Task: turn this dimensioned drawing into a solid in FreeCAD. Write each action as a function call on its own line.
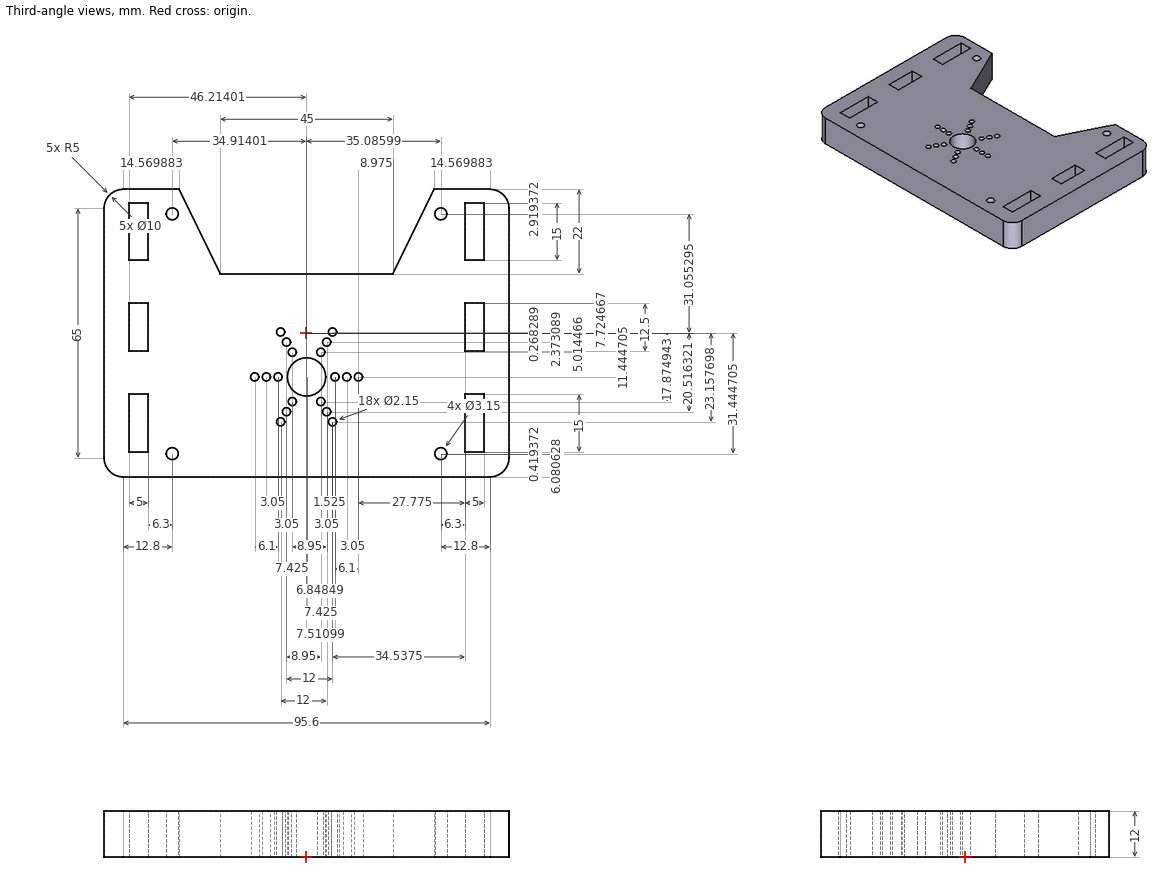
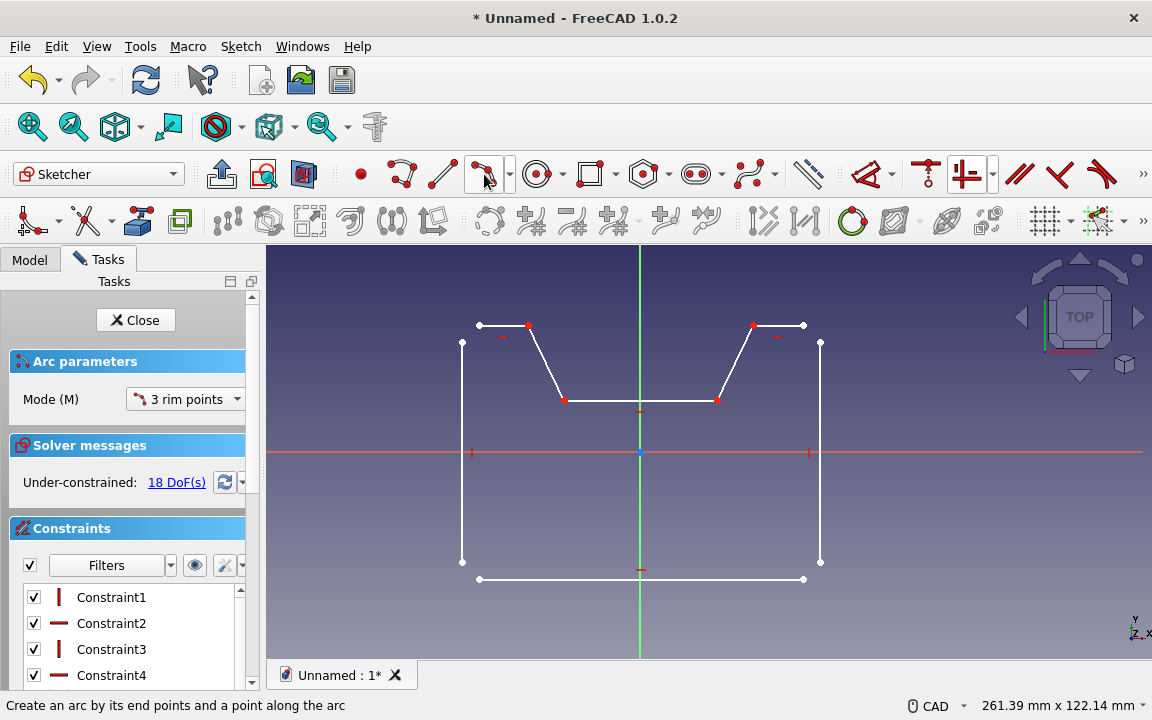
click(462, 563)
click(479, 580)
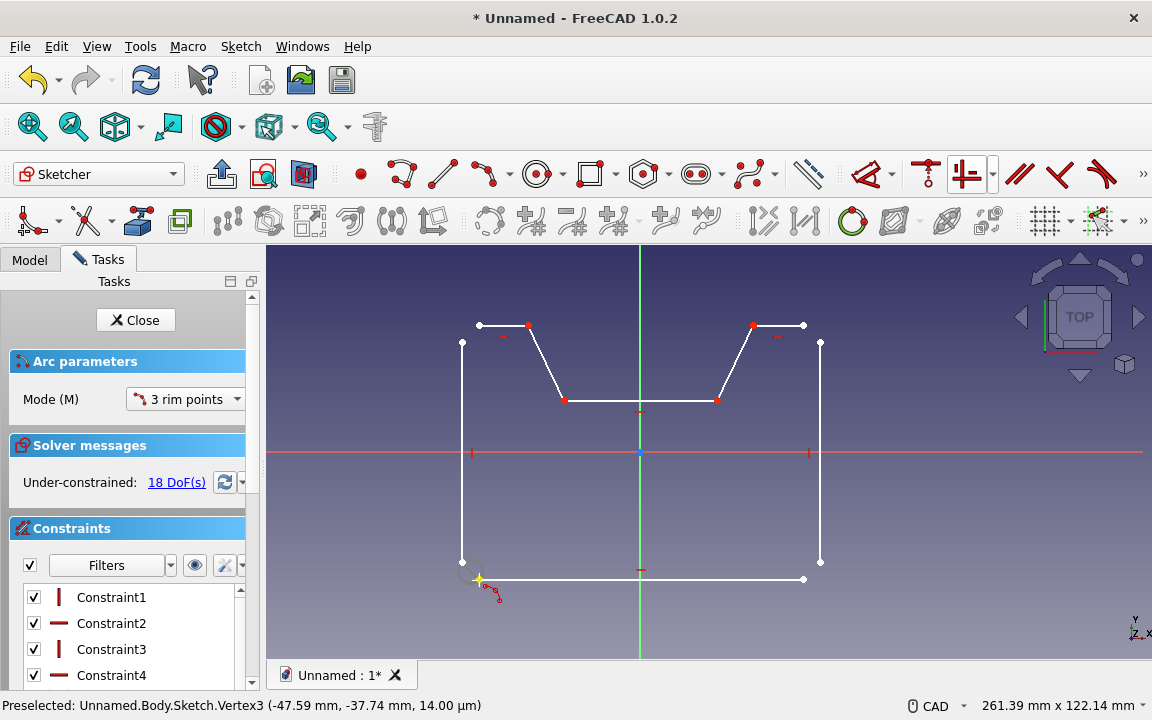
scroll(467, 574, up, 6)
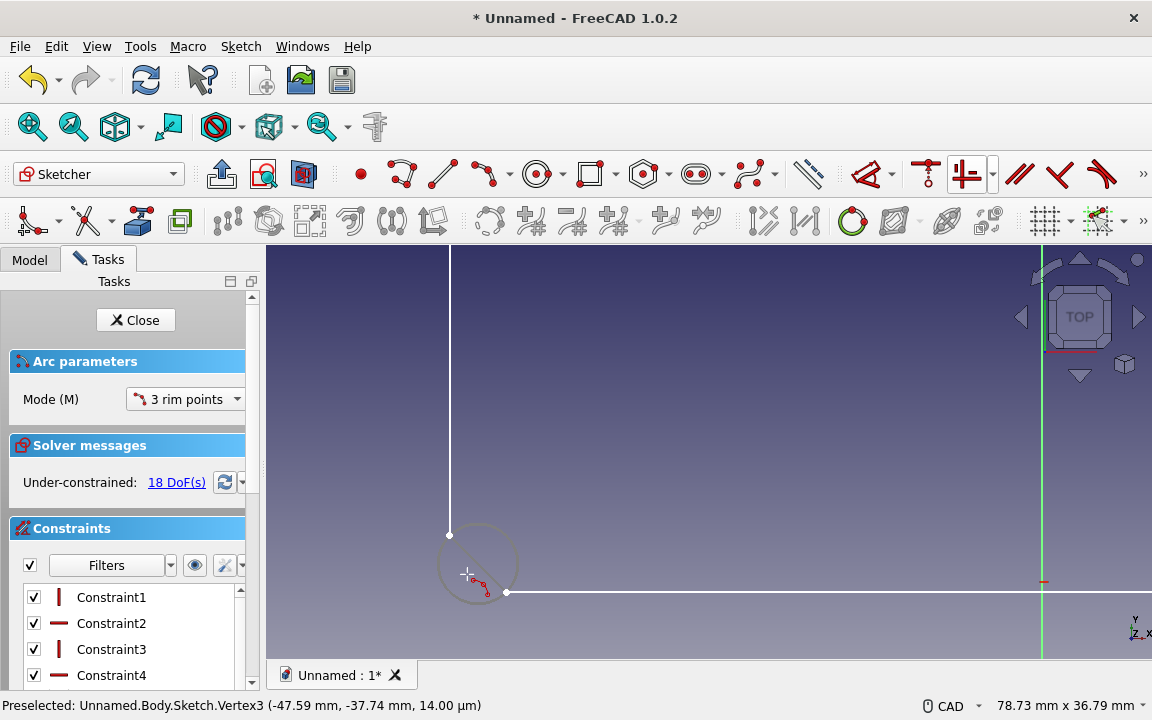
click(465, 573)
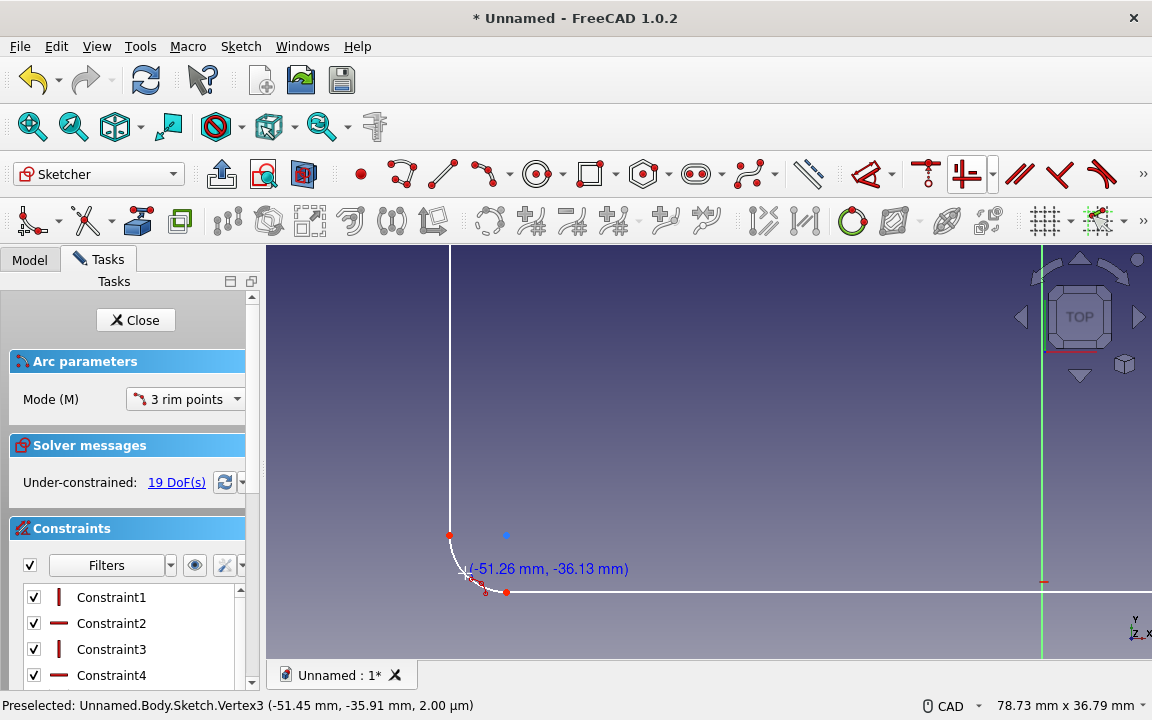
scroll(467, 575, down, 6)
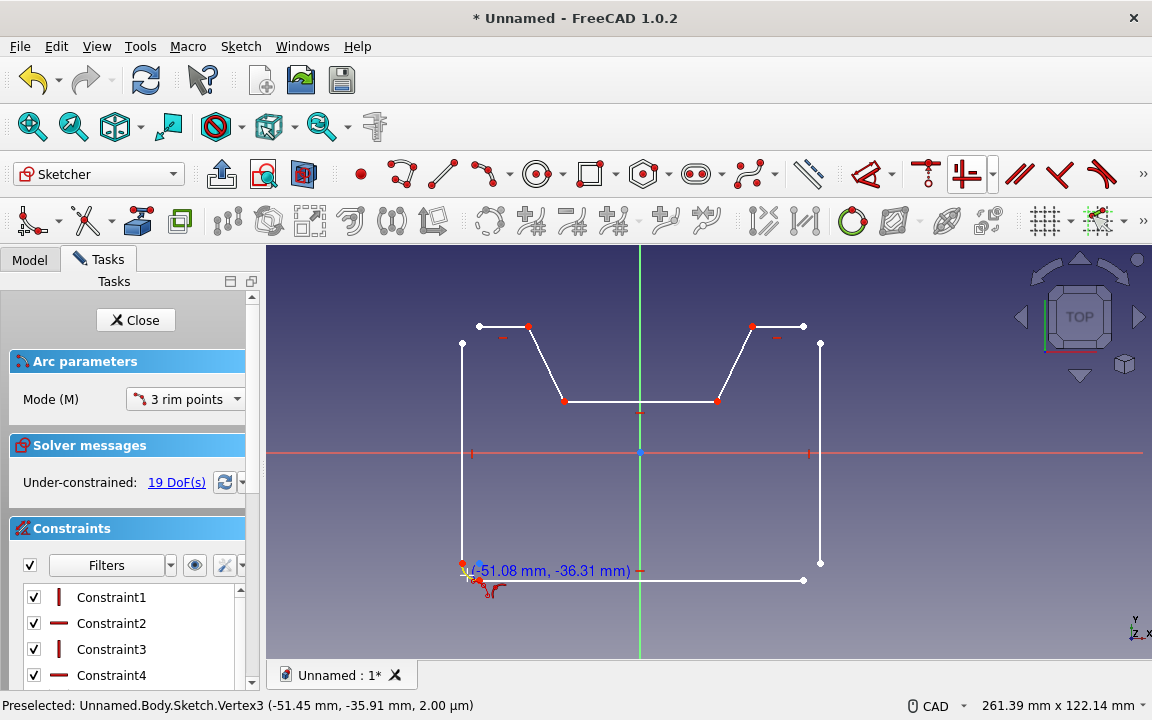
click(803, 581)
click(820, 564)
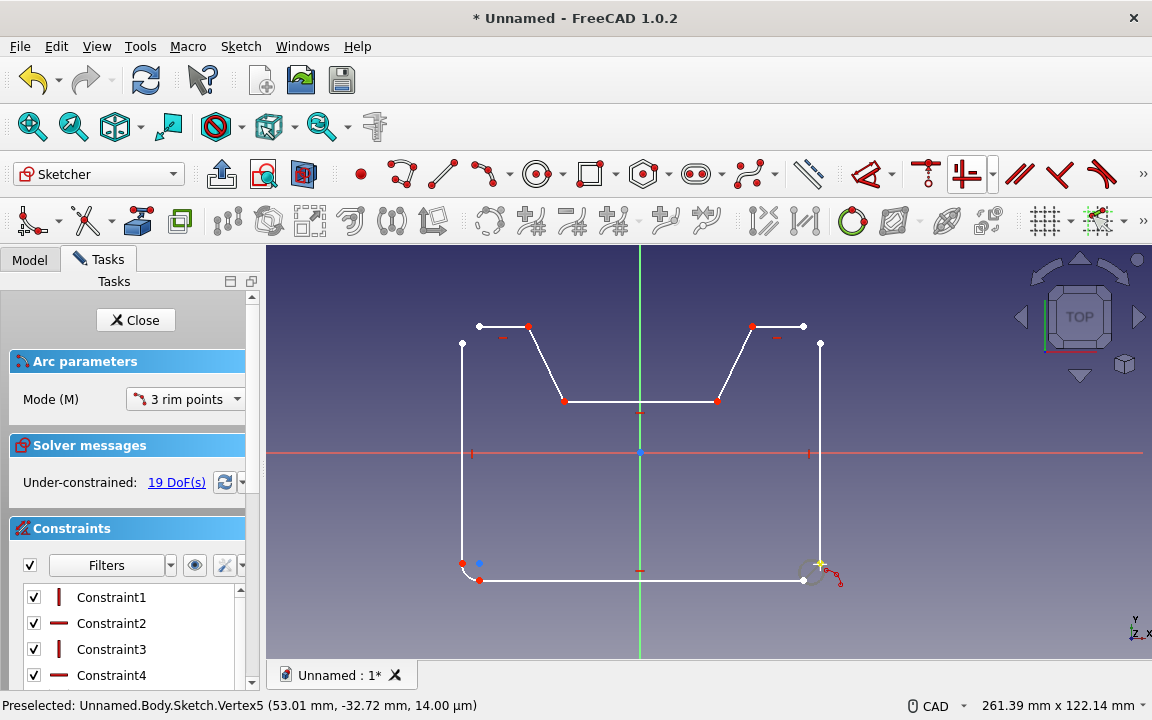
scroll(815, 575, up, 6)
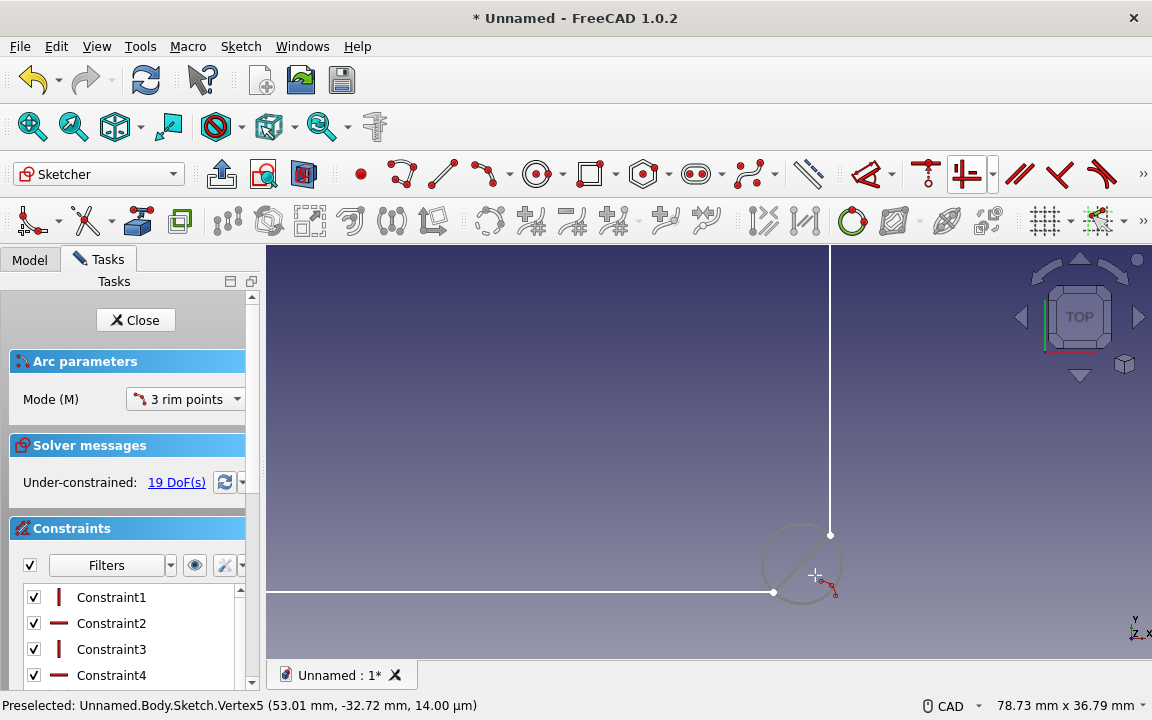
click(812, 573)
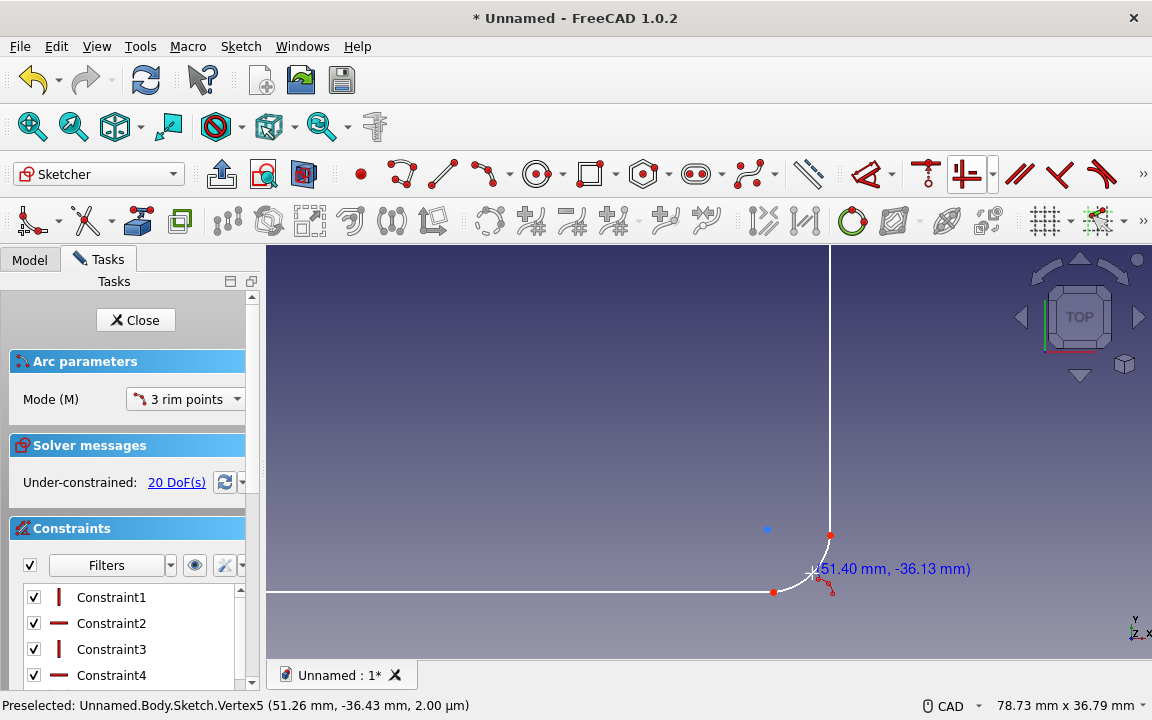
scroll(815, 575, down, 6)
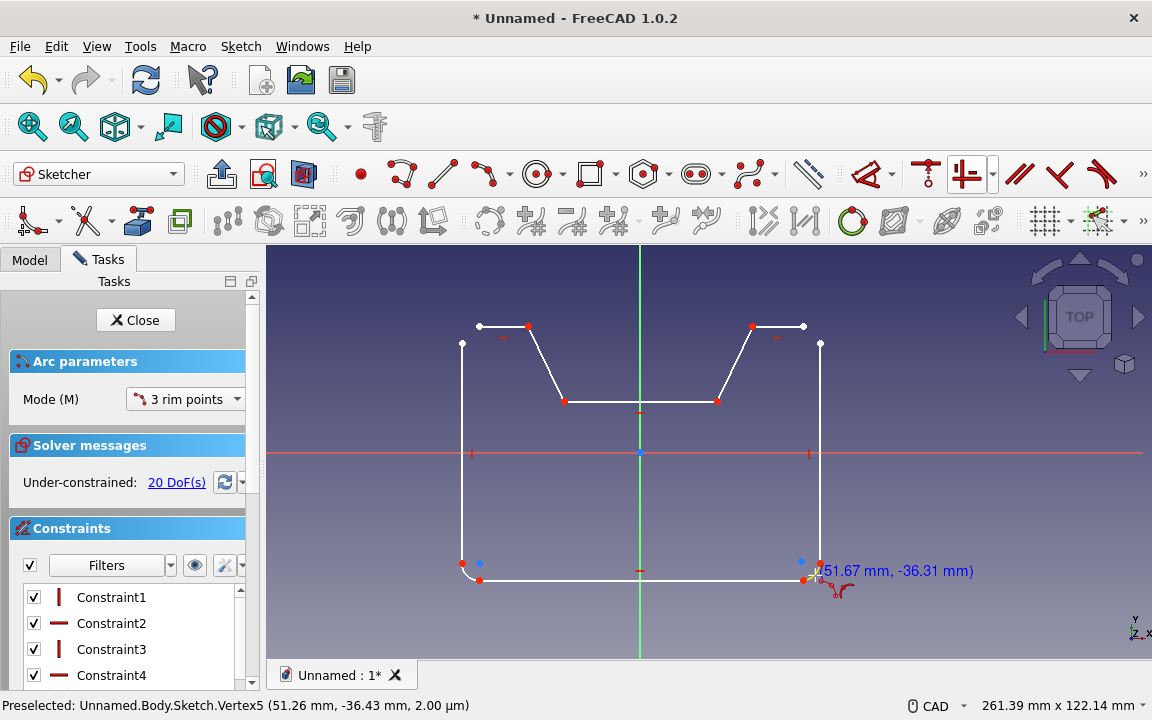
click(820, 344)
click(803, 327)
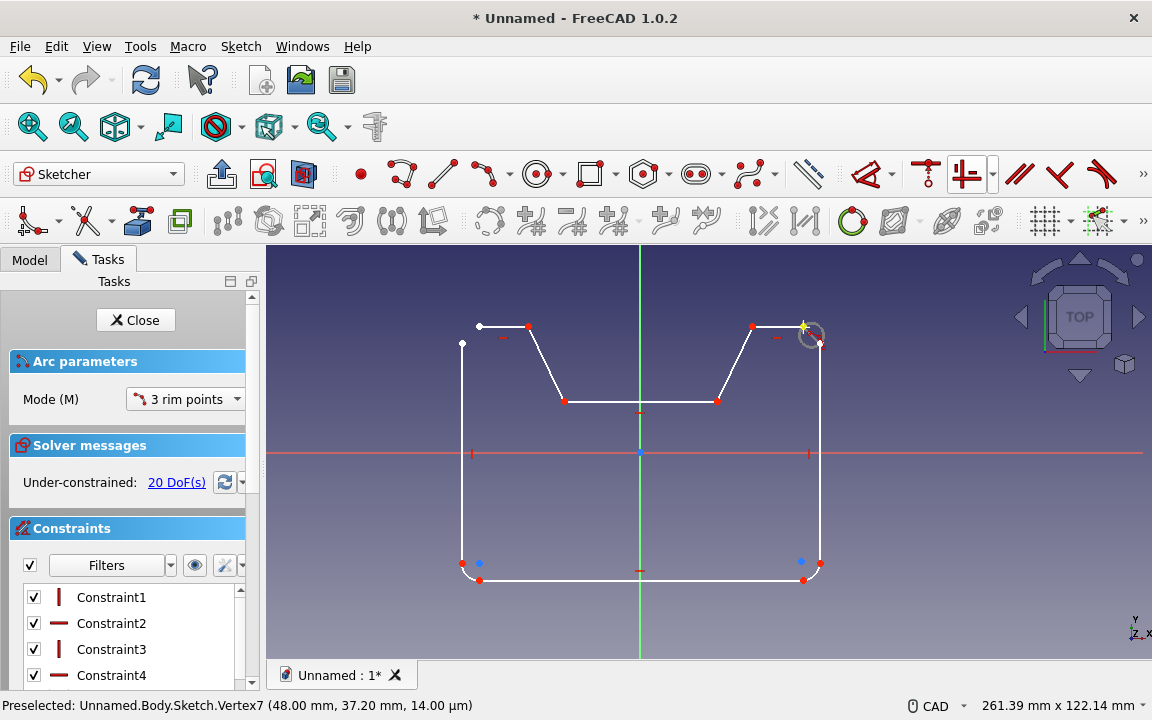
scroll(815, 331, up, 6)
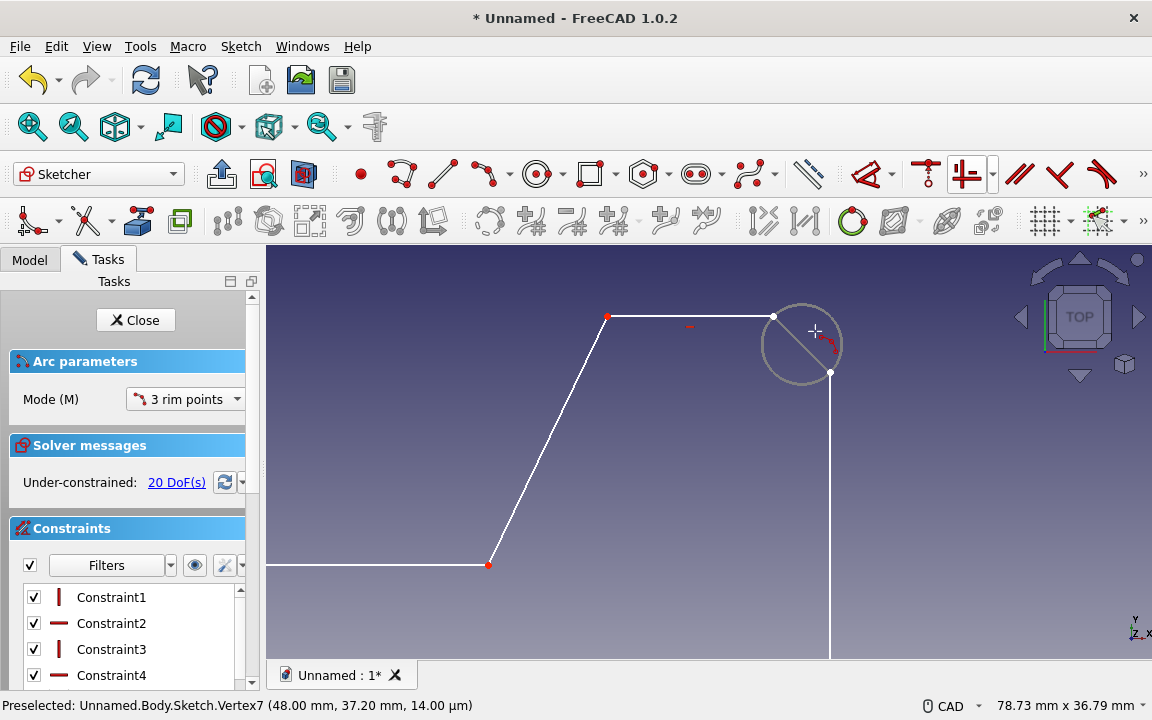
click(812, 330)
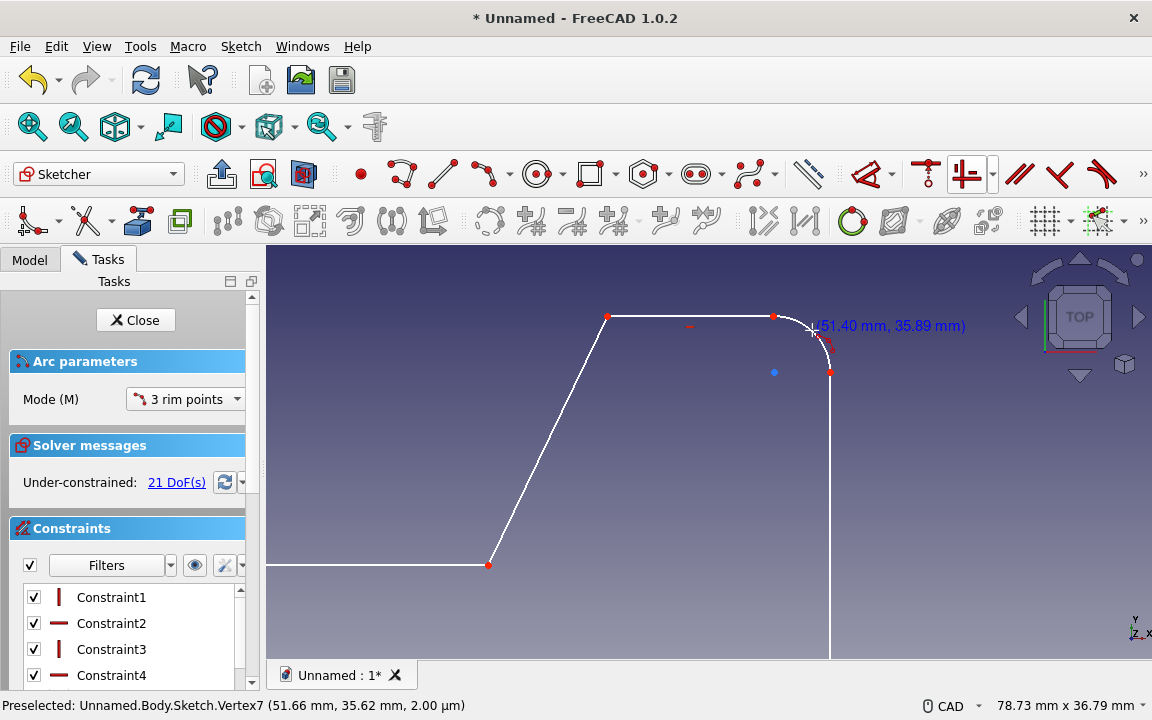
scroll(815, 330, down, 6)